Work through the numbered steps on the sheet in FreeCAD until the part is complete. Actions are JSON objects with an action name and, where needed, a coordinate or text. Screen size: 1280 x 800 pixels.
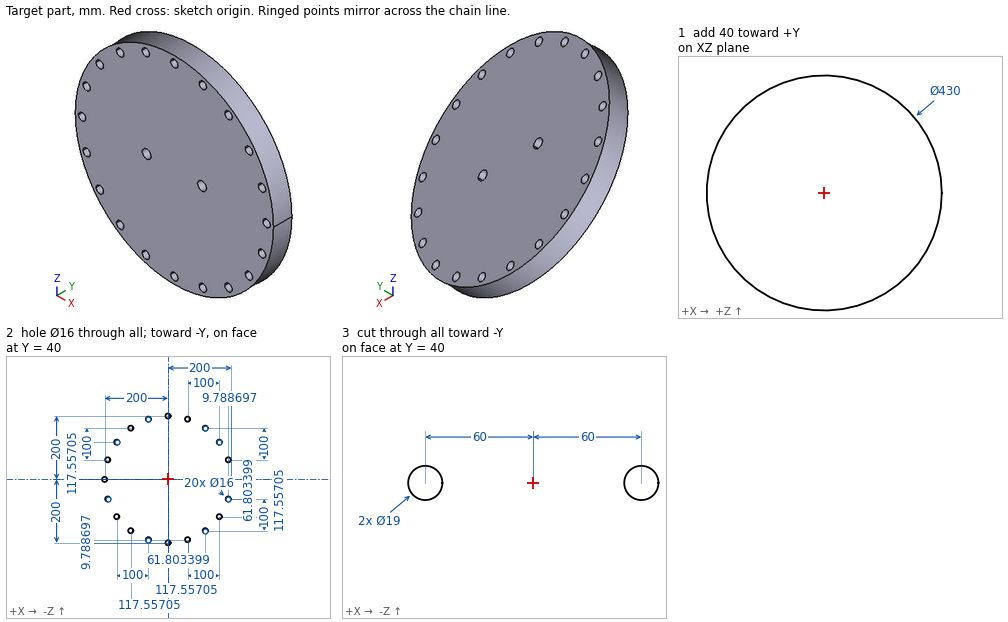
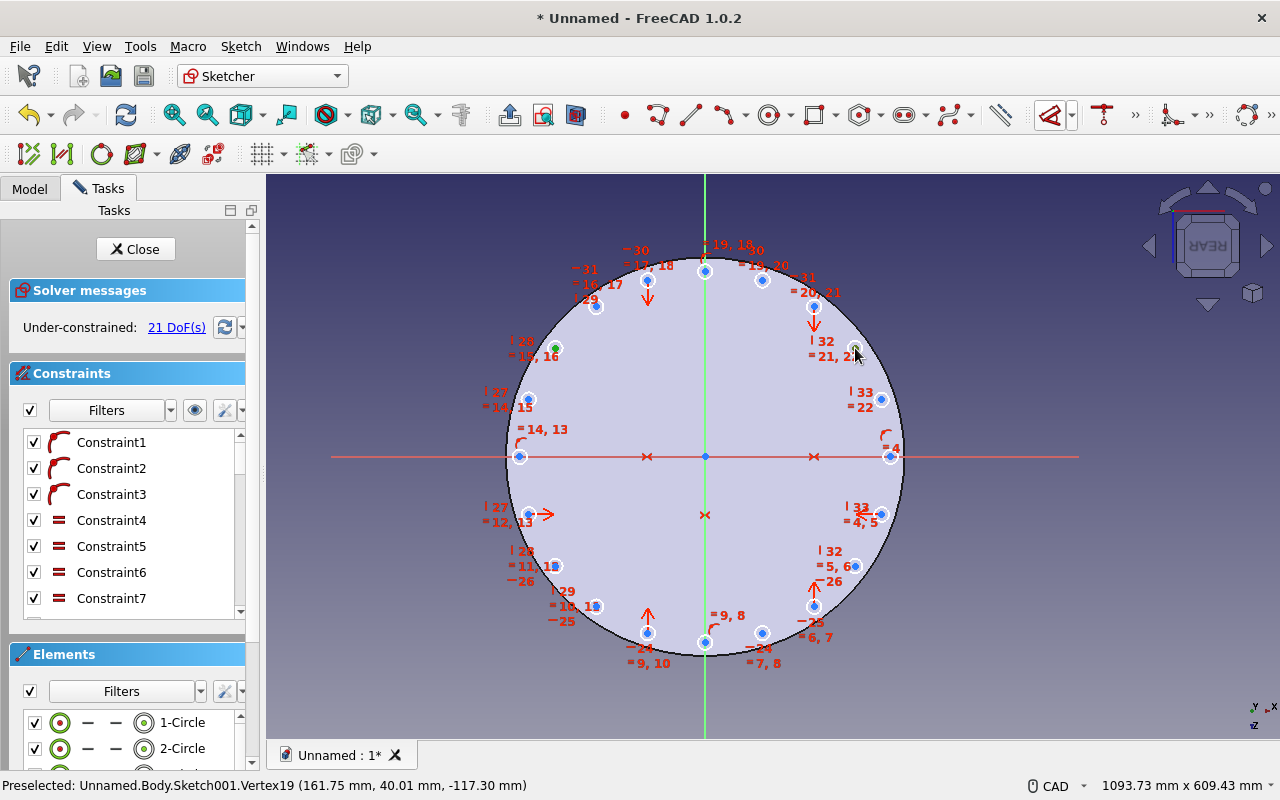
{"action": "left_click", "coordinate": [705, 602]}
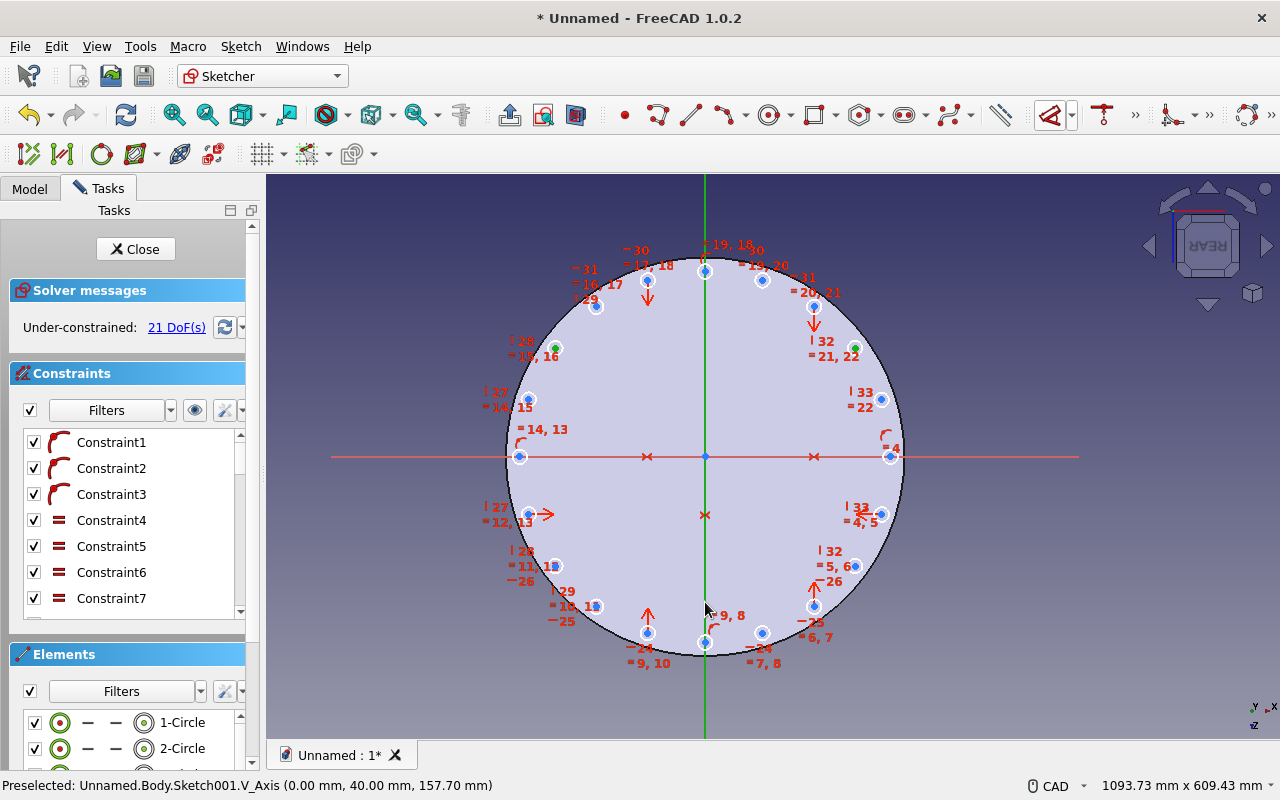
{"action": "key", "text": "s"}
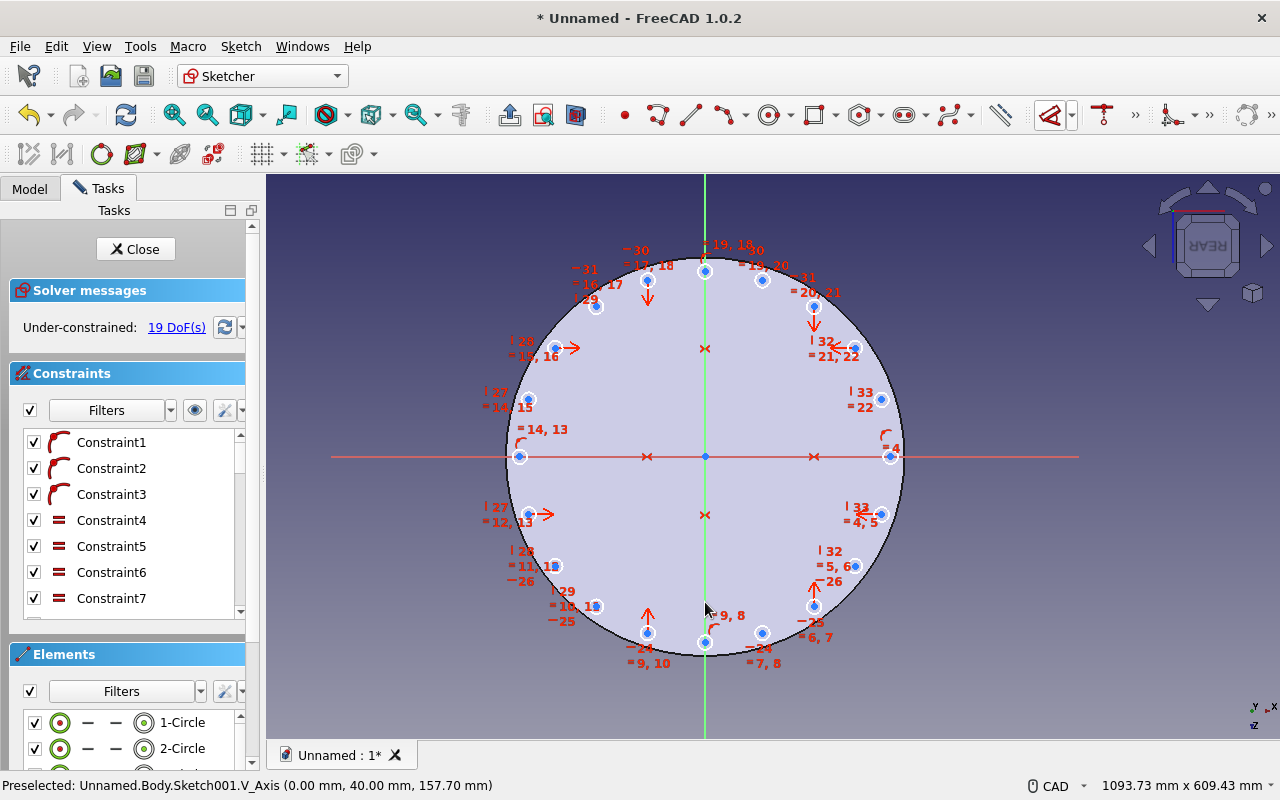
{"action": "key", "text": "d"}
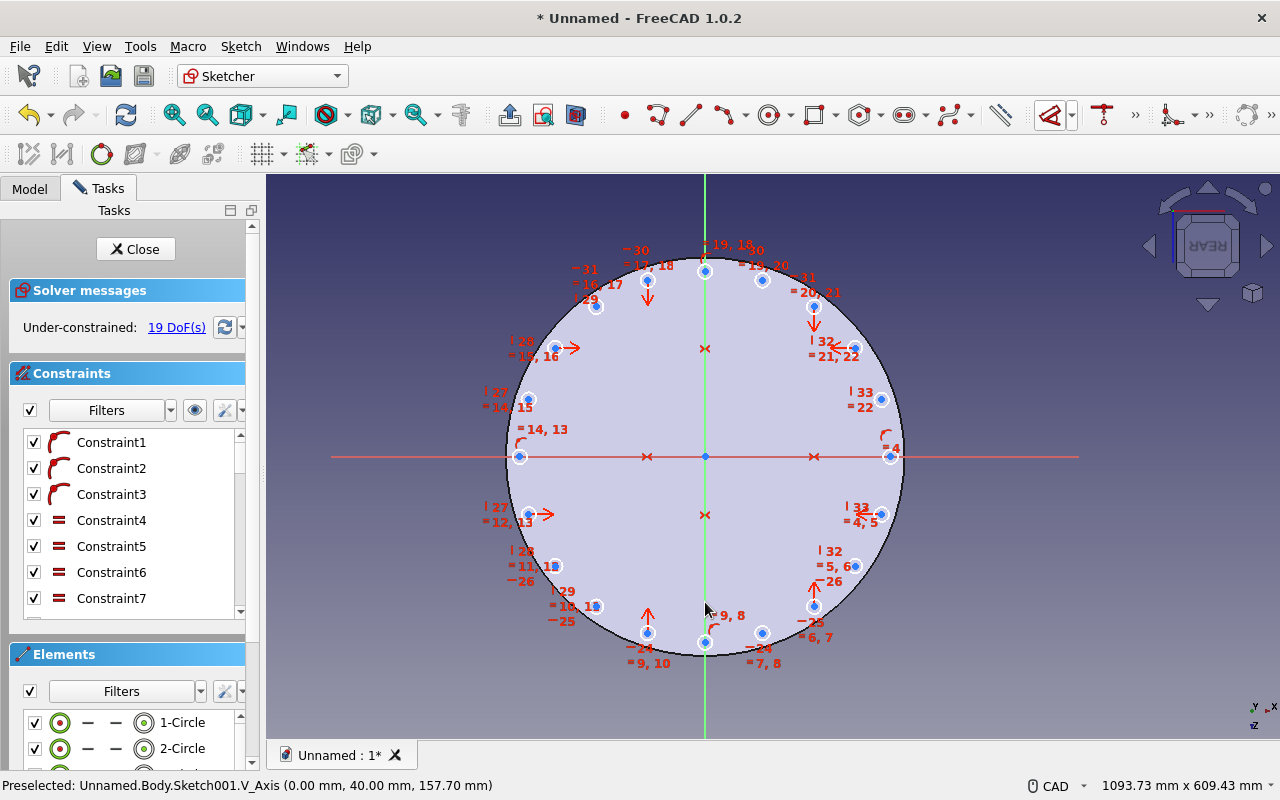
{"action": "scroll", "coordinate": [883, 457], "scroll_direction": "up", "scroll_amount": 5}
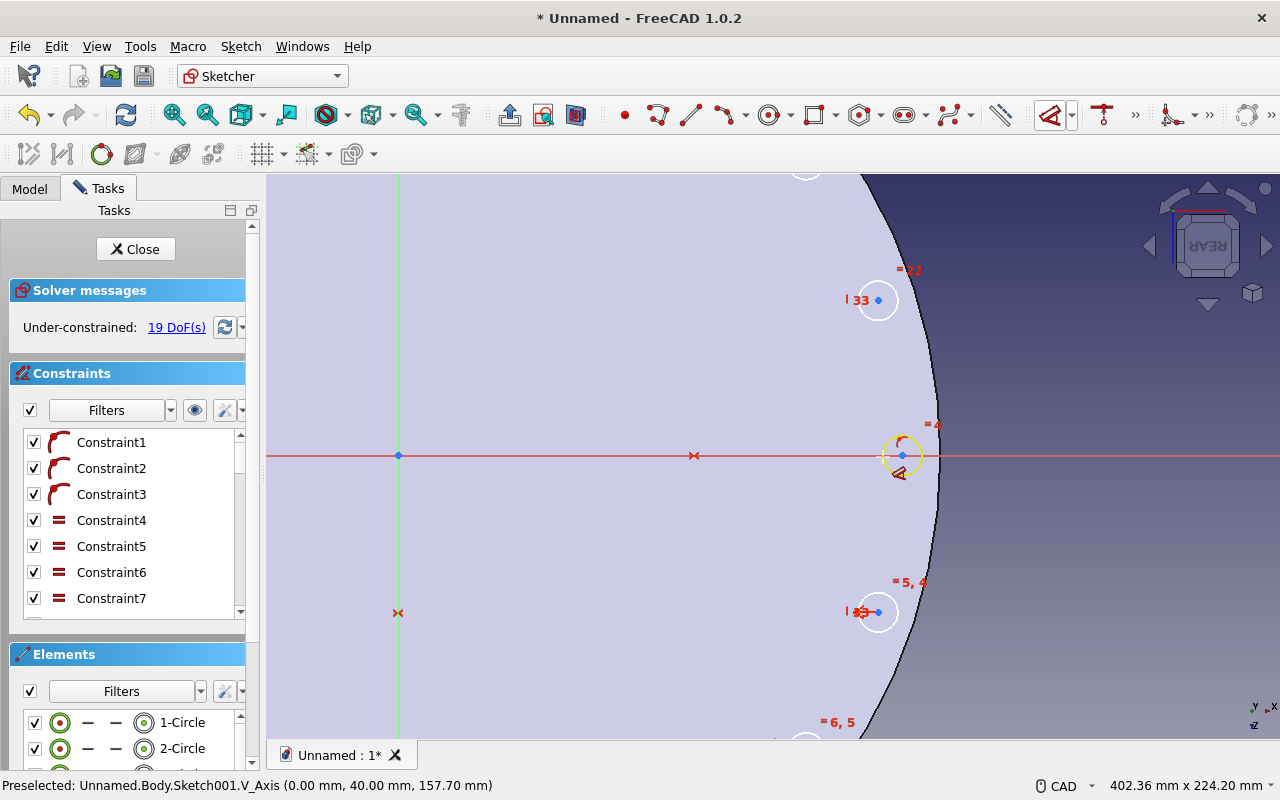
{"action": "left_click", "coordinate": [883, 455]}
{"action": "left_click", "coordinate": [858, 429]}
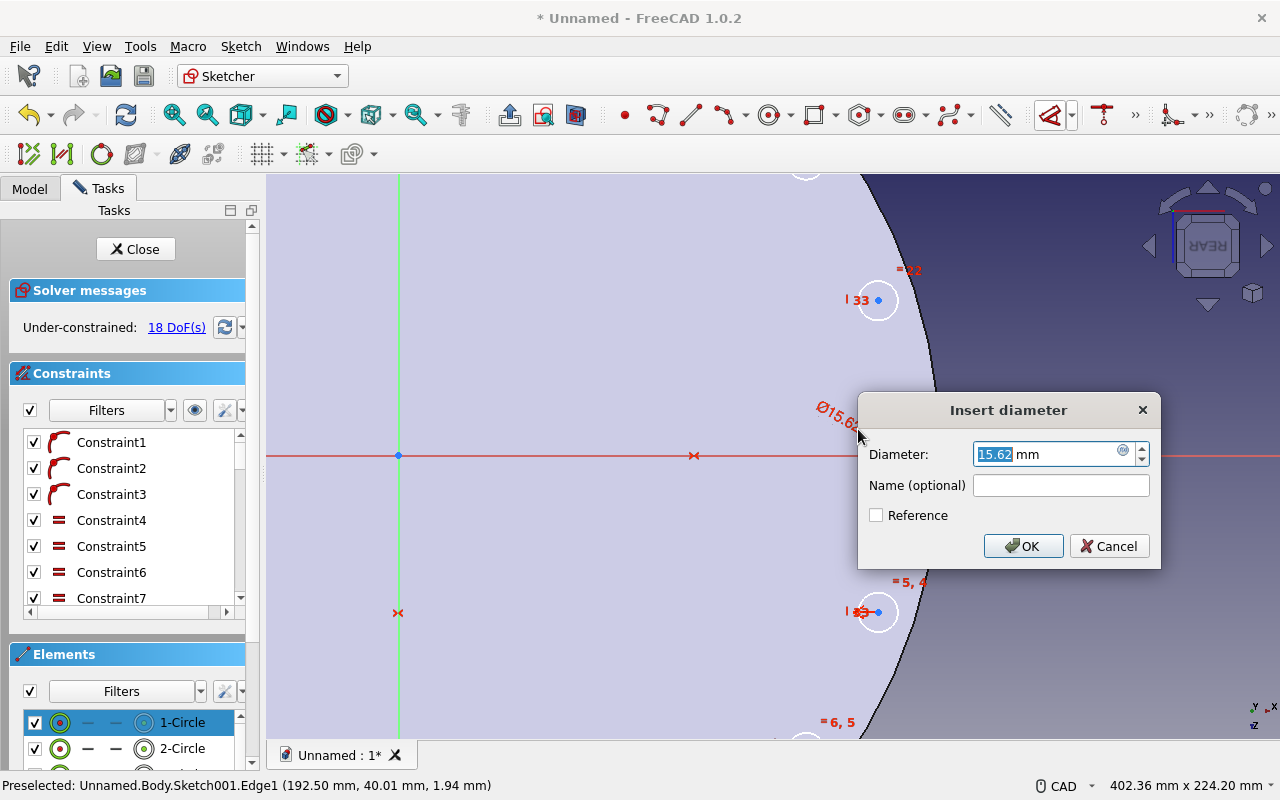
{"action": "type", "text": "16"}
{"action": "key", "text": "Return"}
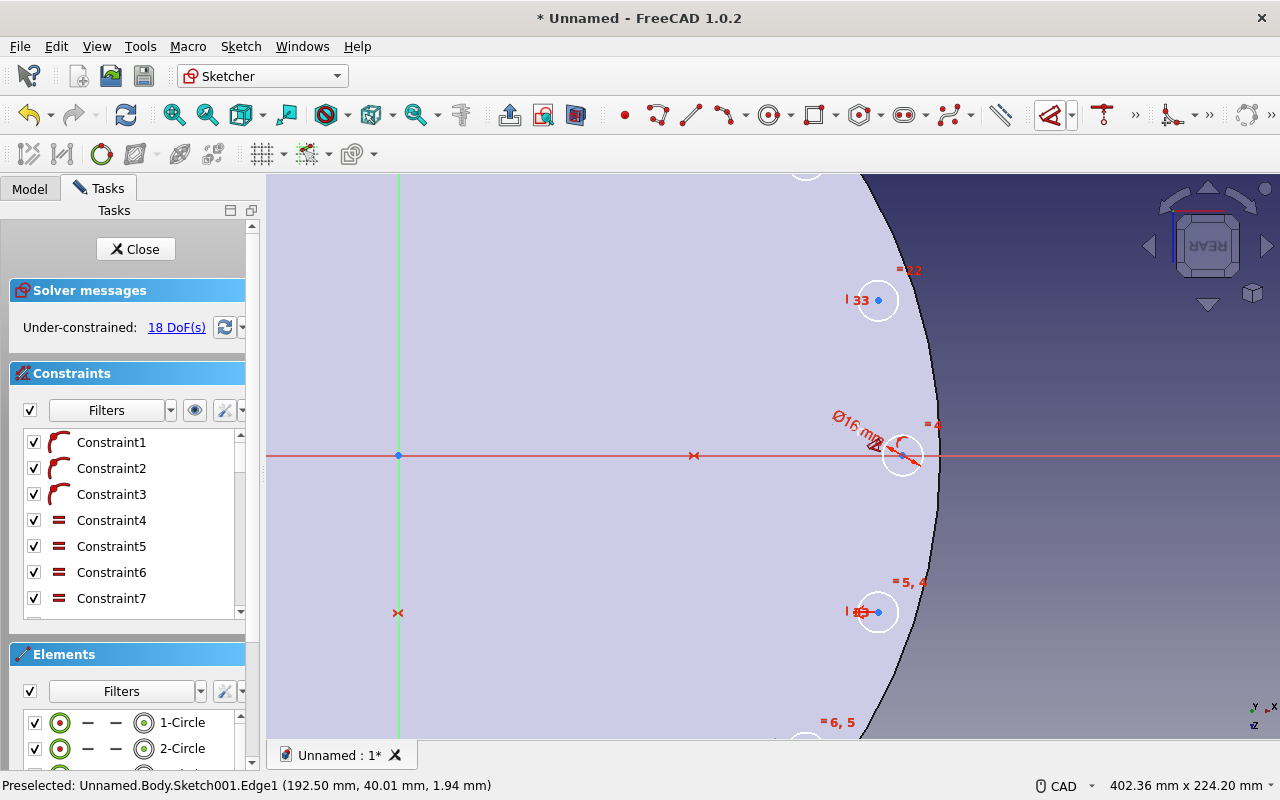
{"action": "left_click", "coordinate": [903, 456]}
{"action": "left_click", "coordinate": [651, 490]}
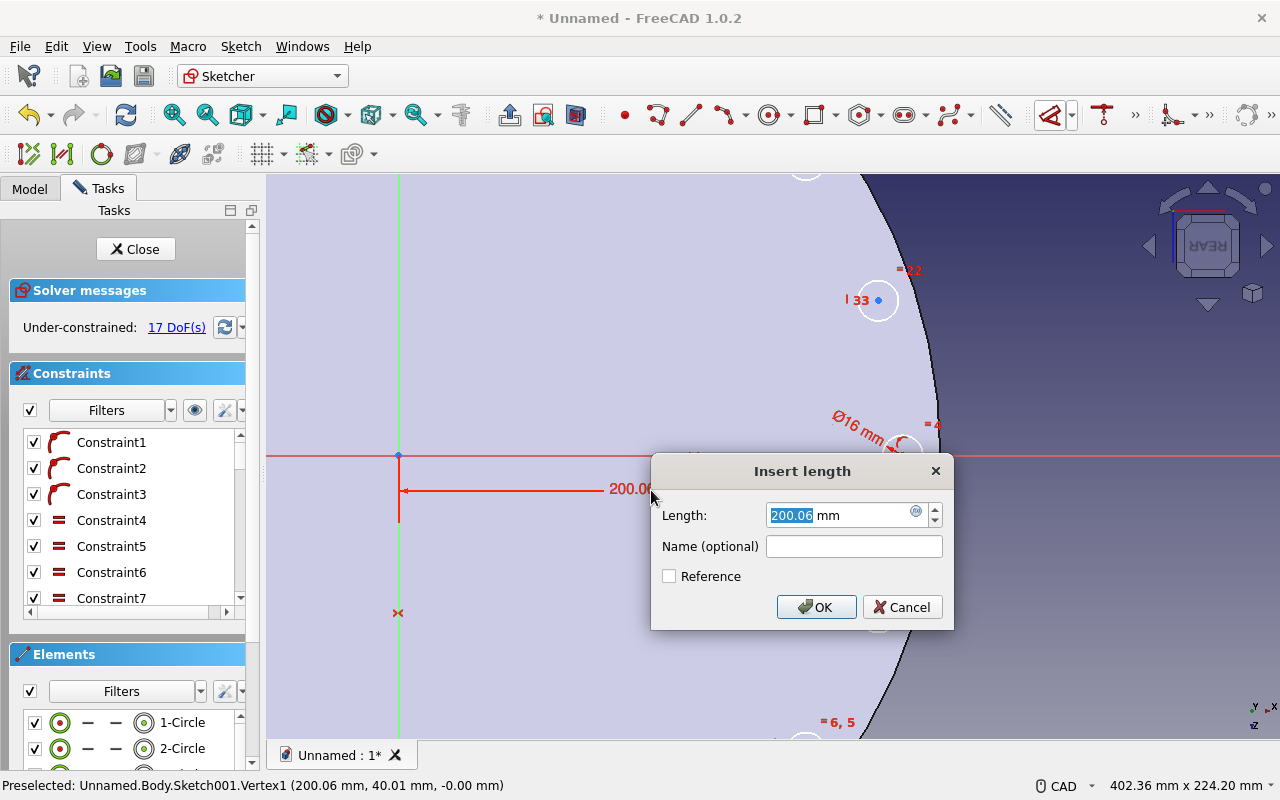
{"action": "type", "text": "200"}
{"action": "key", "text": "Return"}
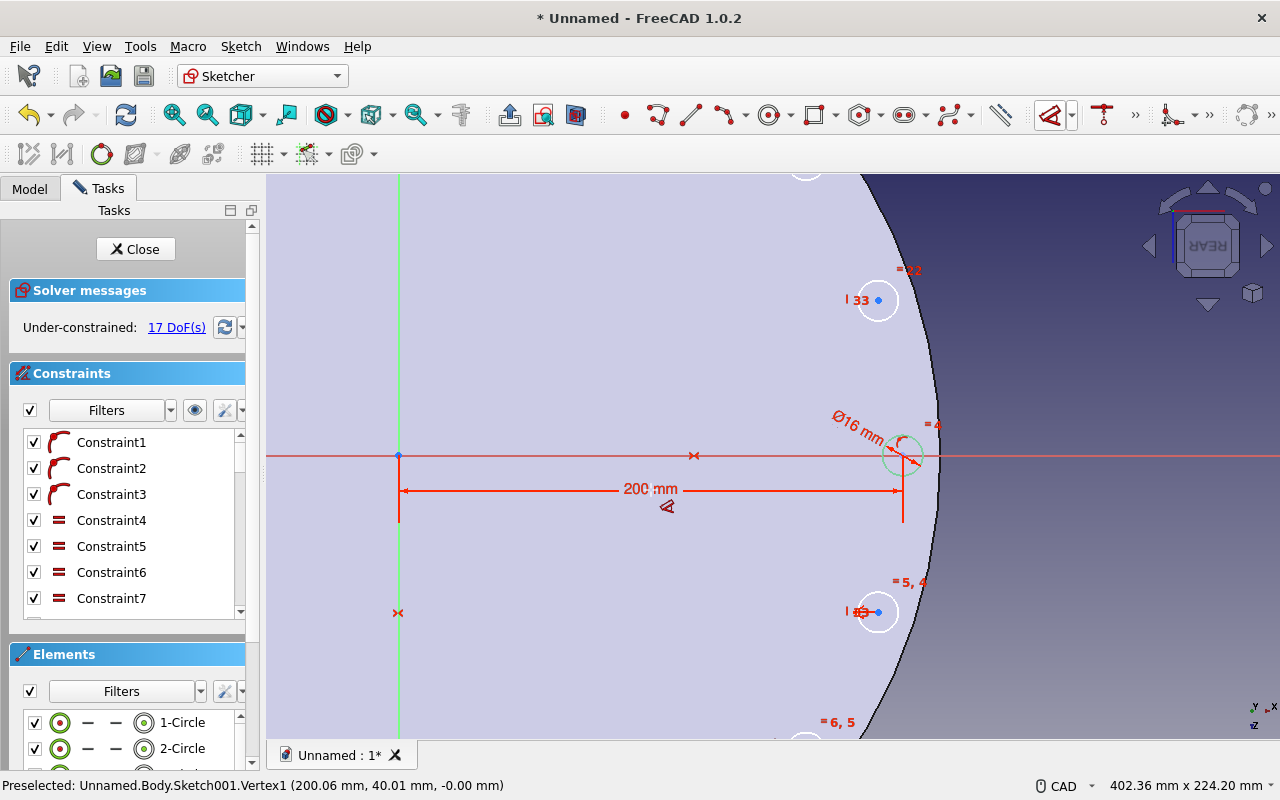
{"action": "scroll", "coordinate": [883, 457], "scroll_direction": "down", "scroll_amount": 5}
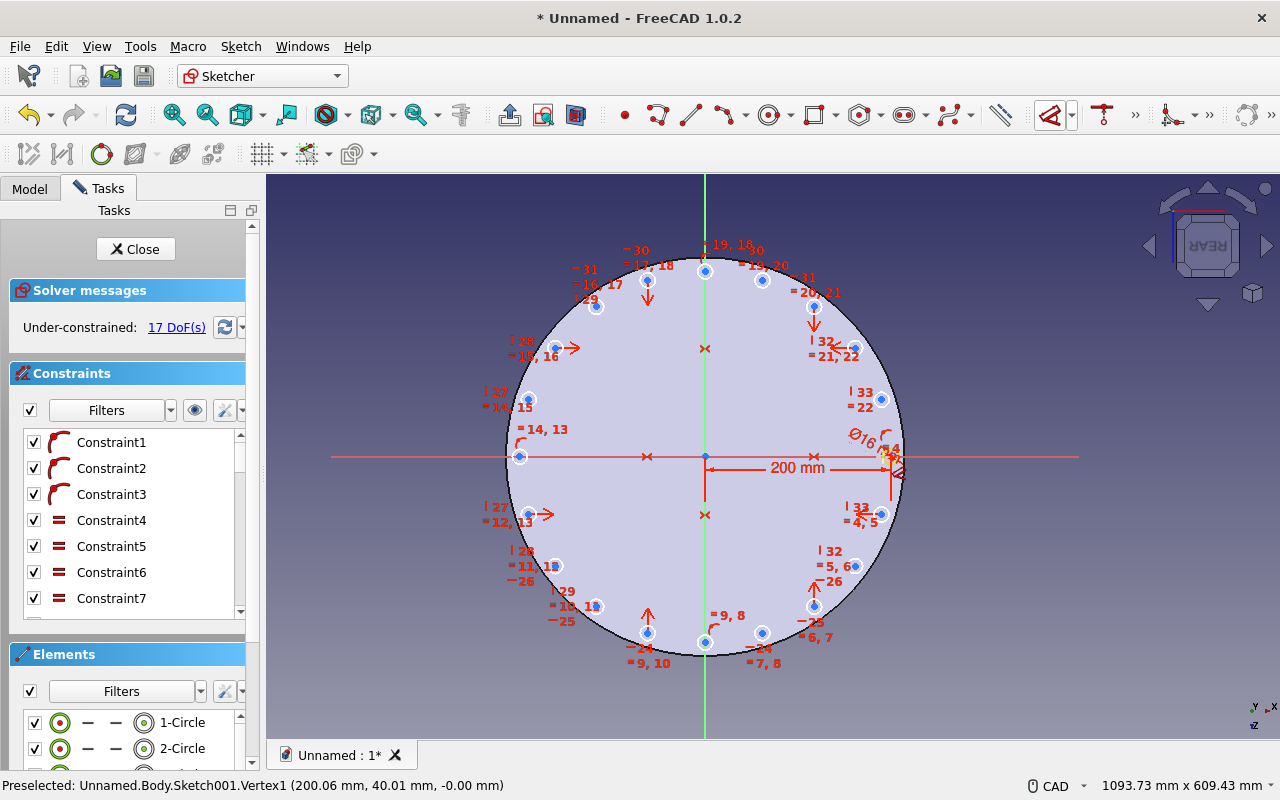
{"action": "left_click", "coordinate": [705, 643]}
{"action": "left_click", "coordinate": [739, 550]}